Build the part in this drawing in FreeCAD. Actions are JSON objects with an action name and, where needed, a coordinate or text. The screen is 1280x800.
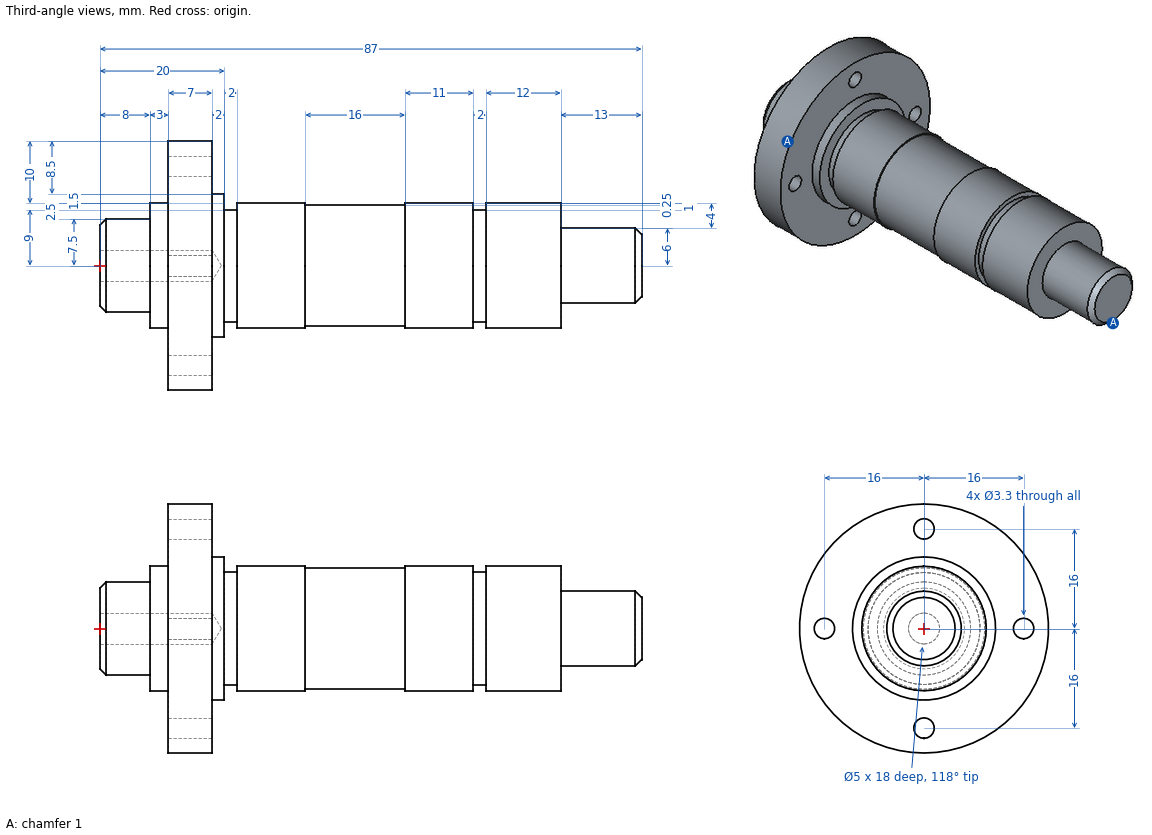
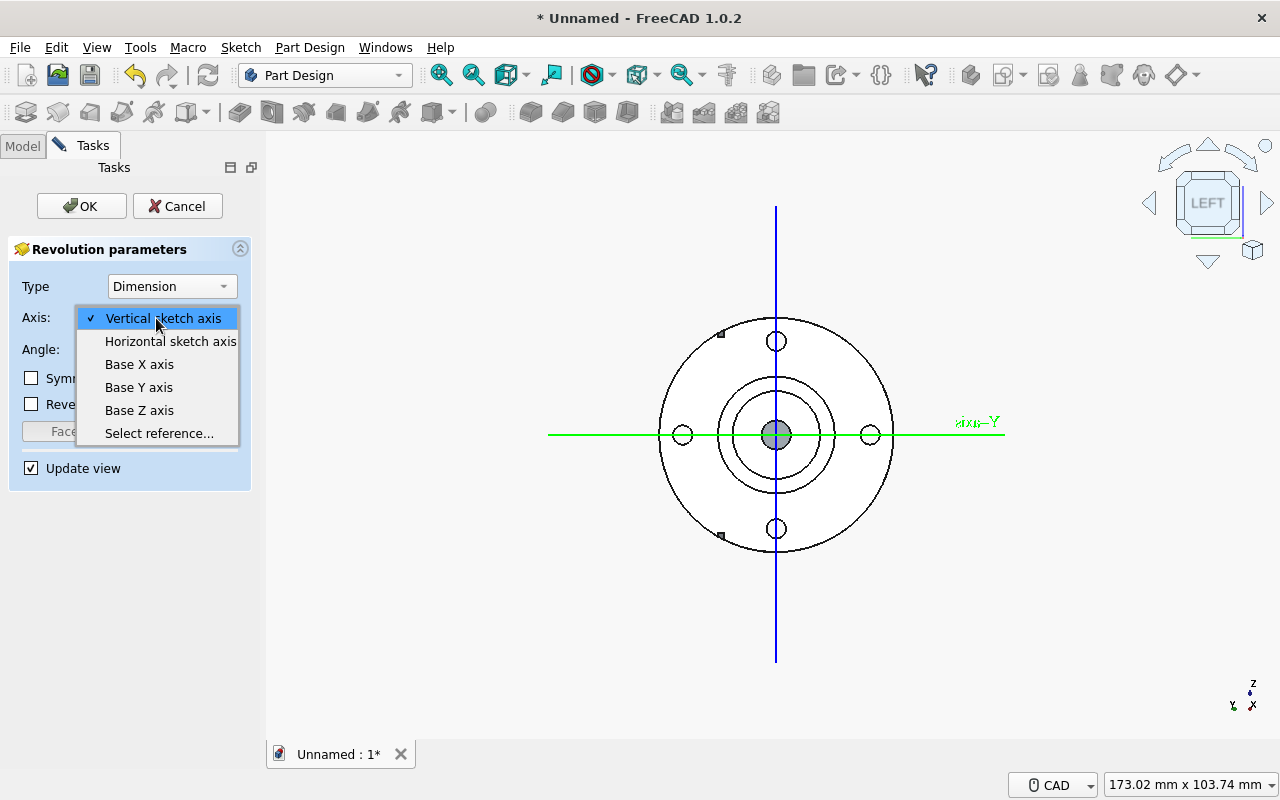
{"action": "left_click", "coordinate": [156, 342]}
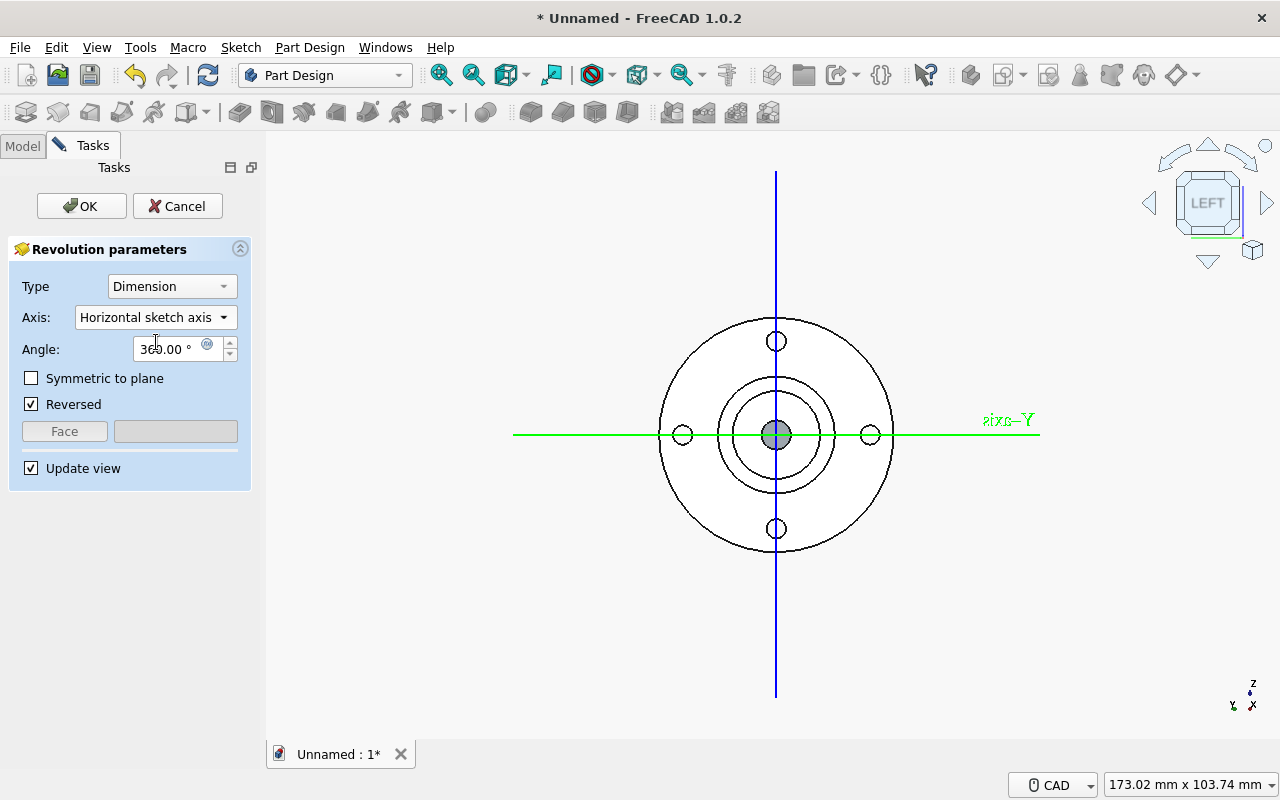
{"action": "left_click", "coordinate": [82, 206]}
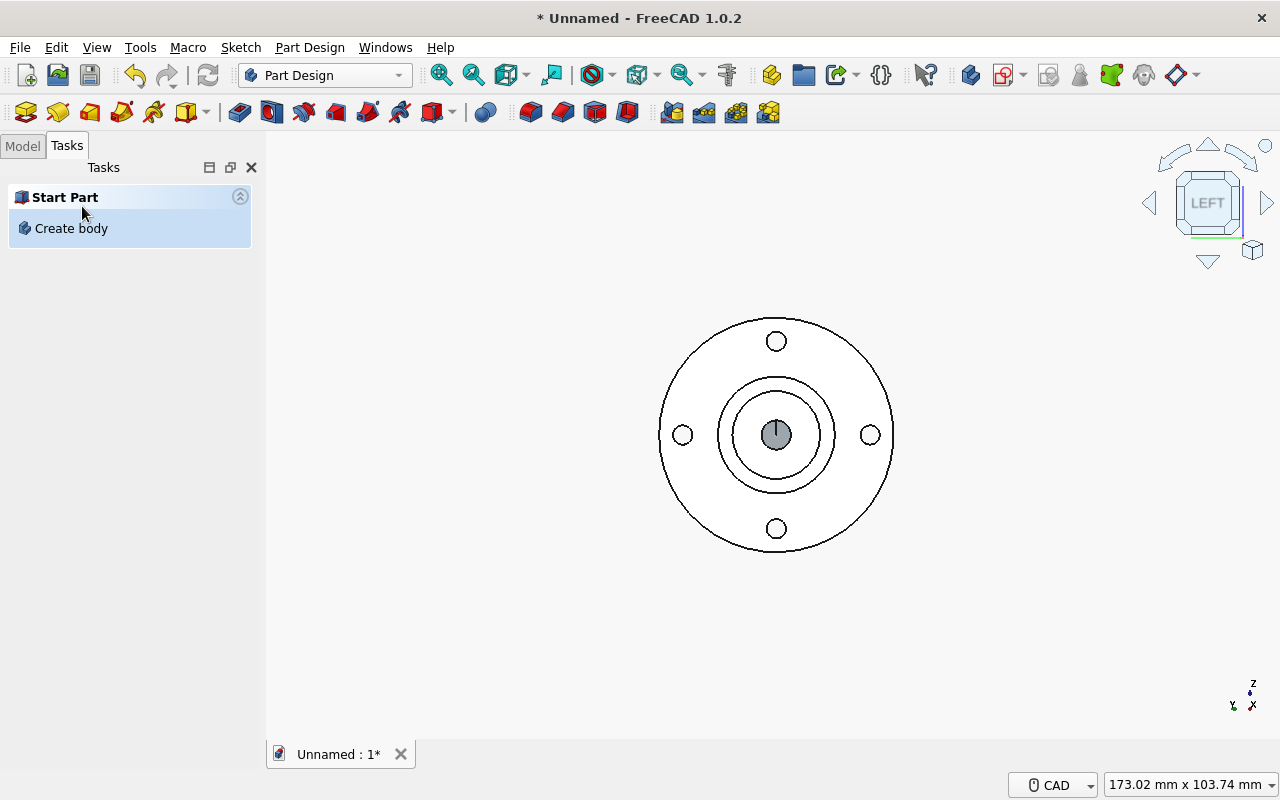
{"action": "left_click", "coordinate": [442, 76]}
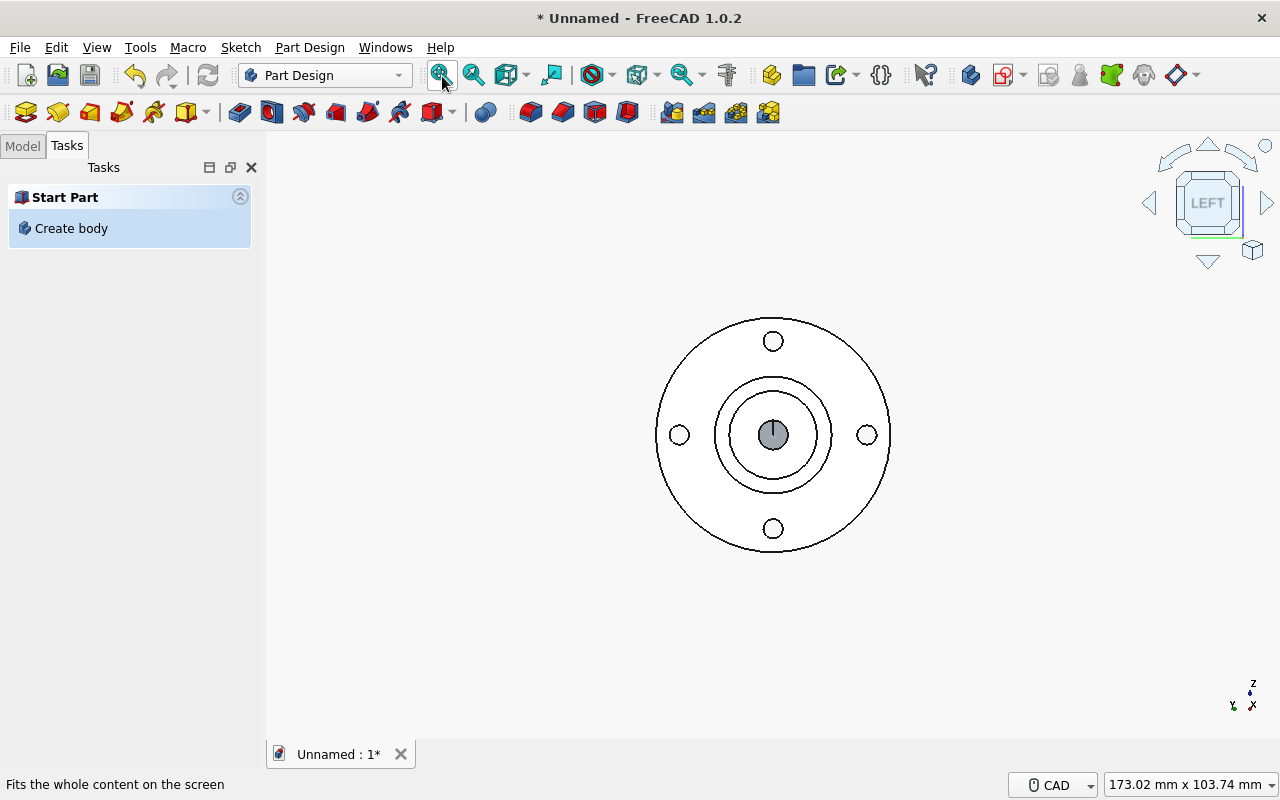
{"action": "left_click", "coordinate": [817, 434]}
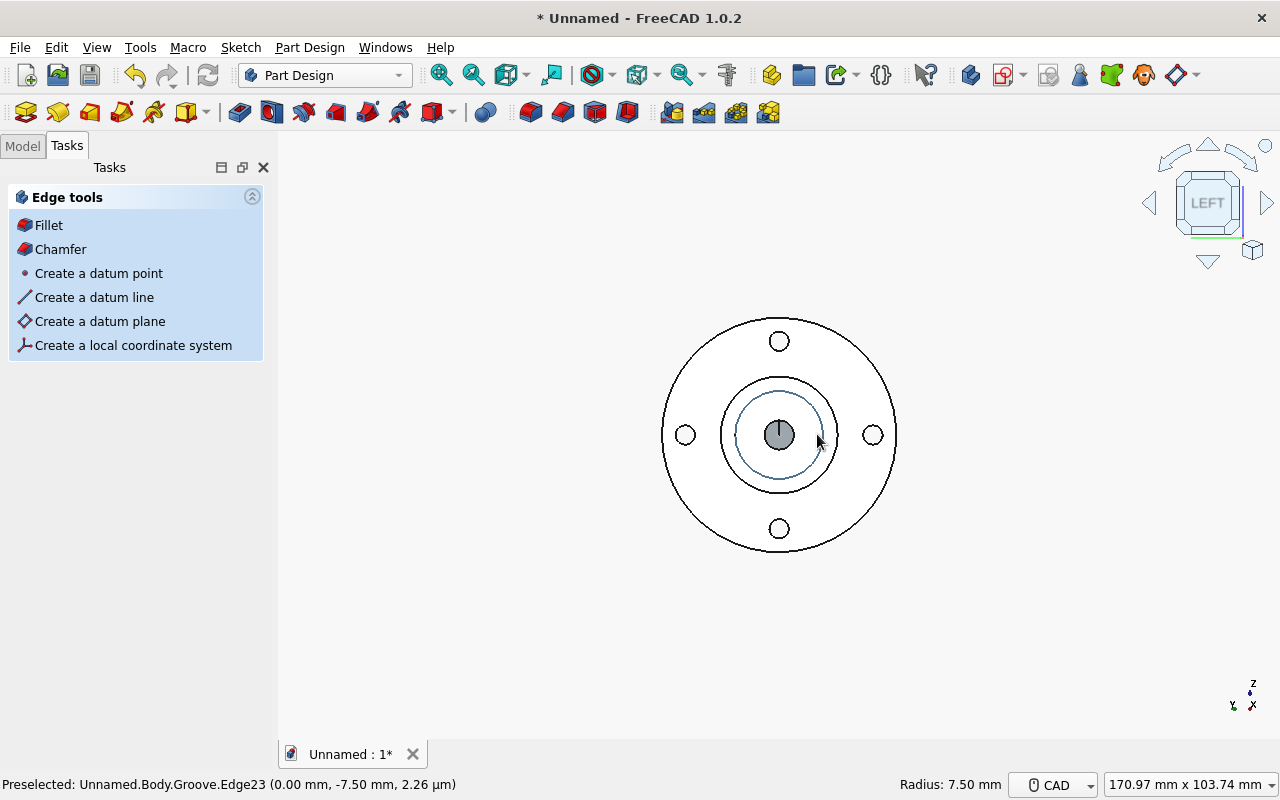
{"action": "key", "text": "0"}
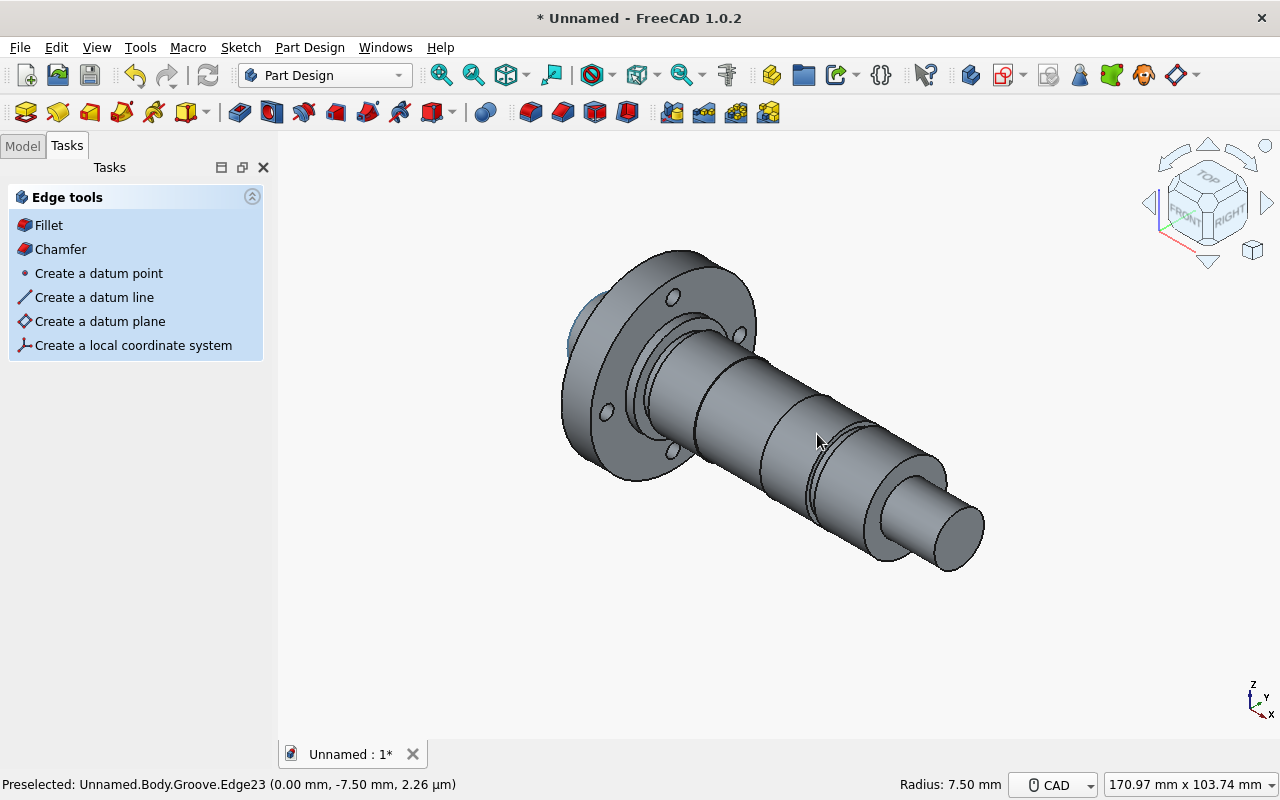
{"action": "left_click", "coordinate": [934, 552], "text": "ctrl"}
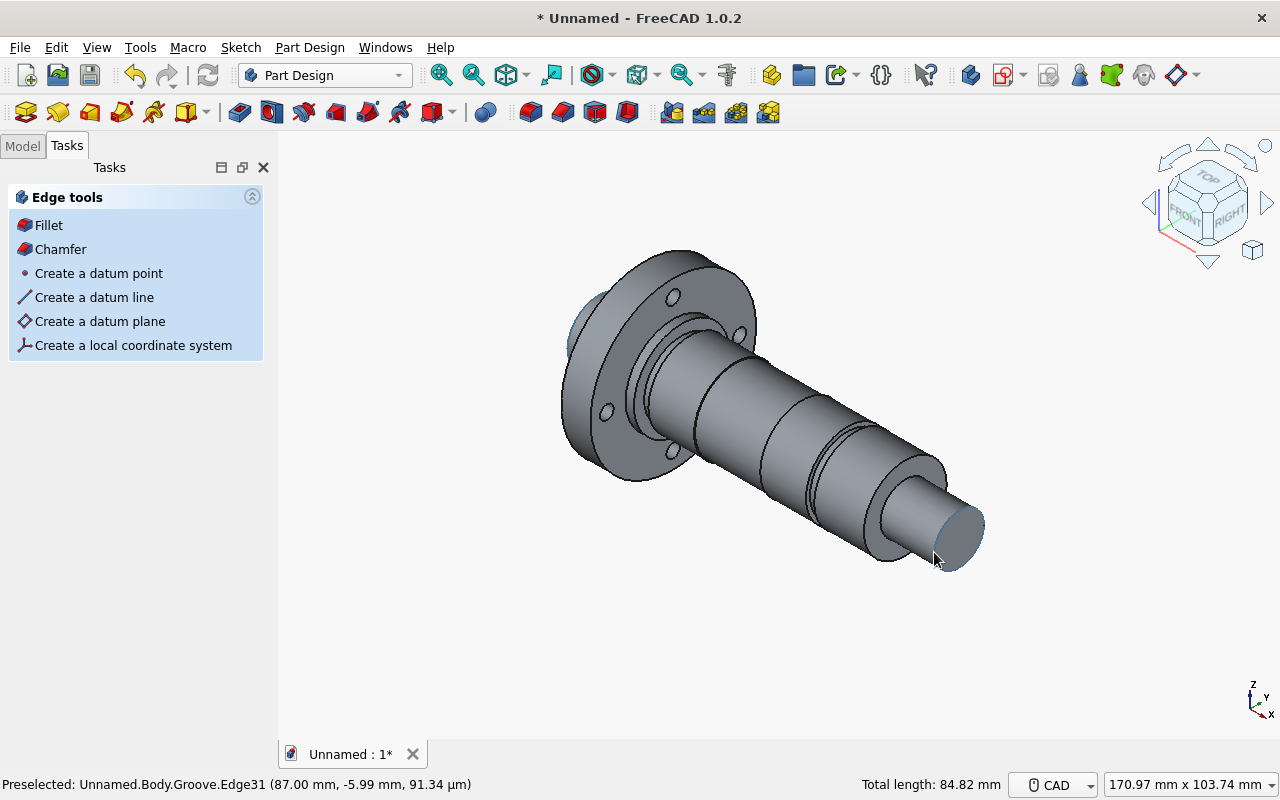
{"action": "left_click", "coordinate": [564, 112]}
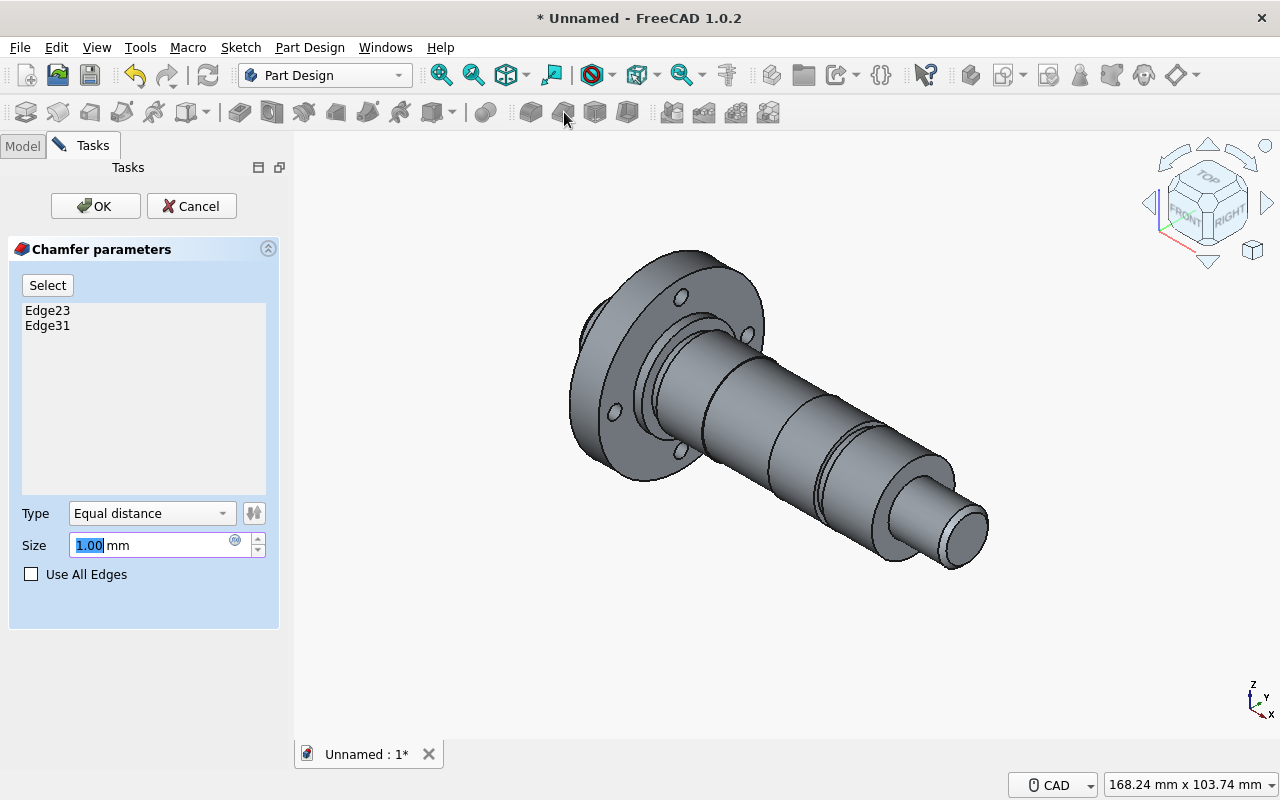
{"action": "type", "text": "1"}
{"action": "key", "text": "Tab"}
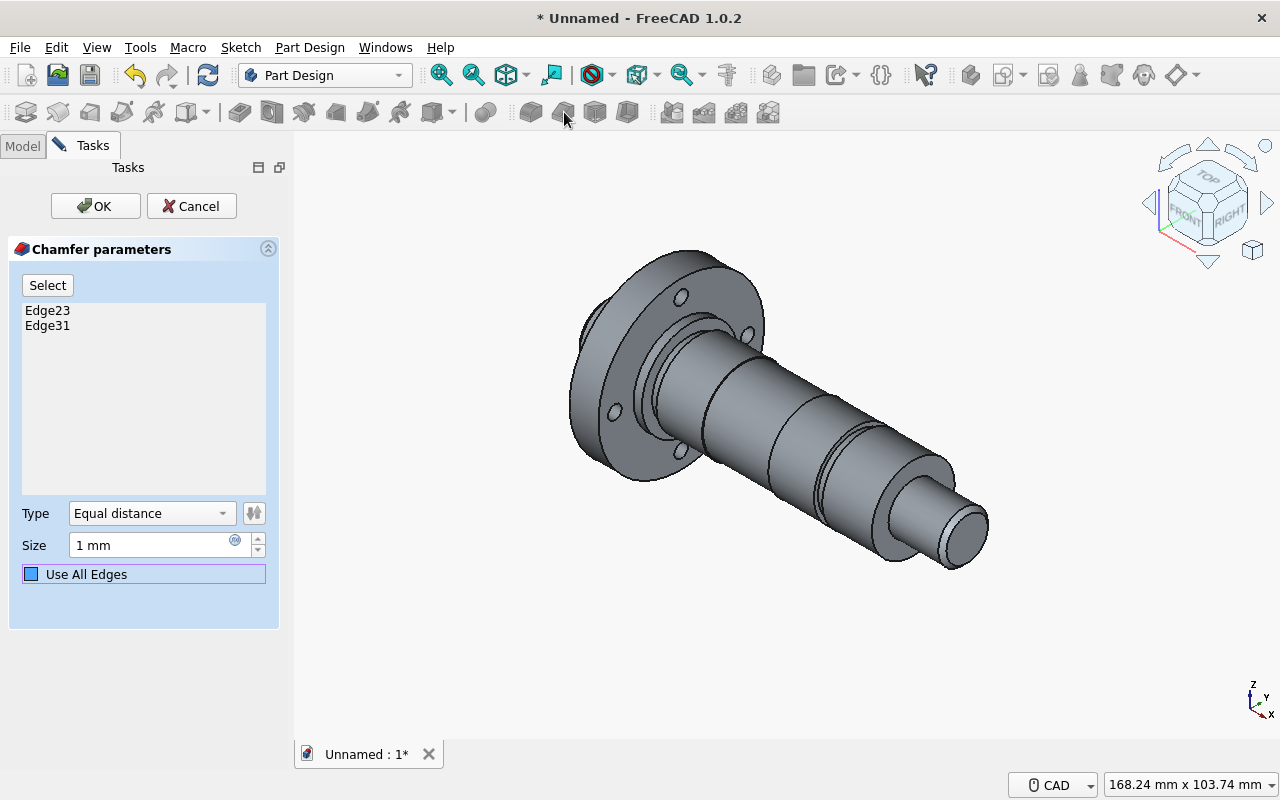
{"action": "left_click", "coordinate": [96, 206]}